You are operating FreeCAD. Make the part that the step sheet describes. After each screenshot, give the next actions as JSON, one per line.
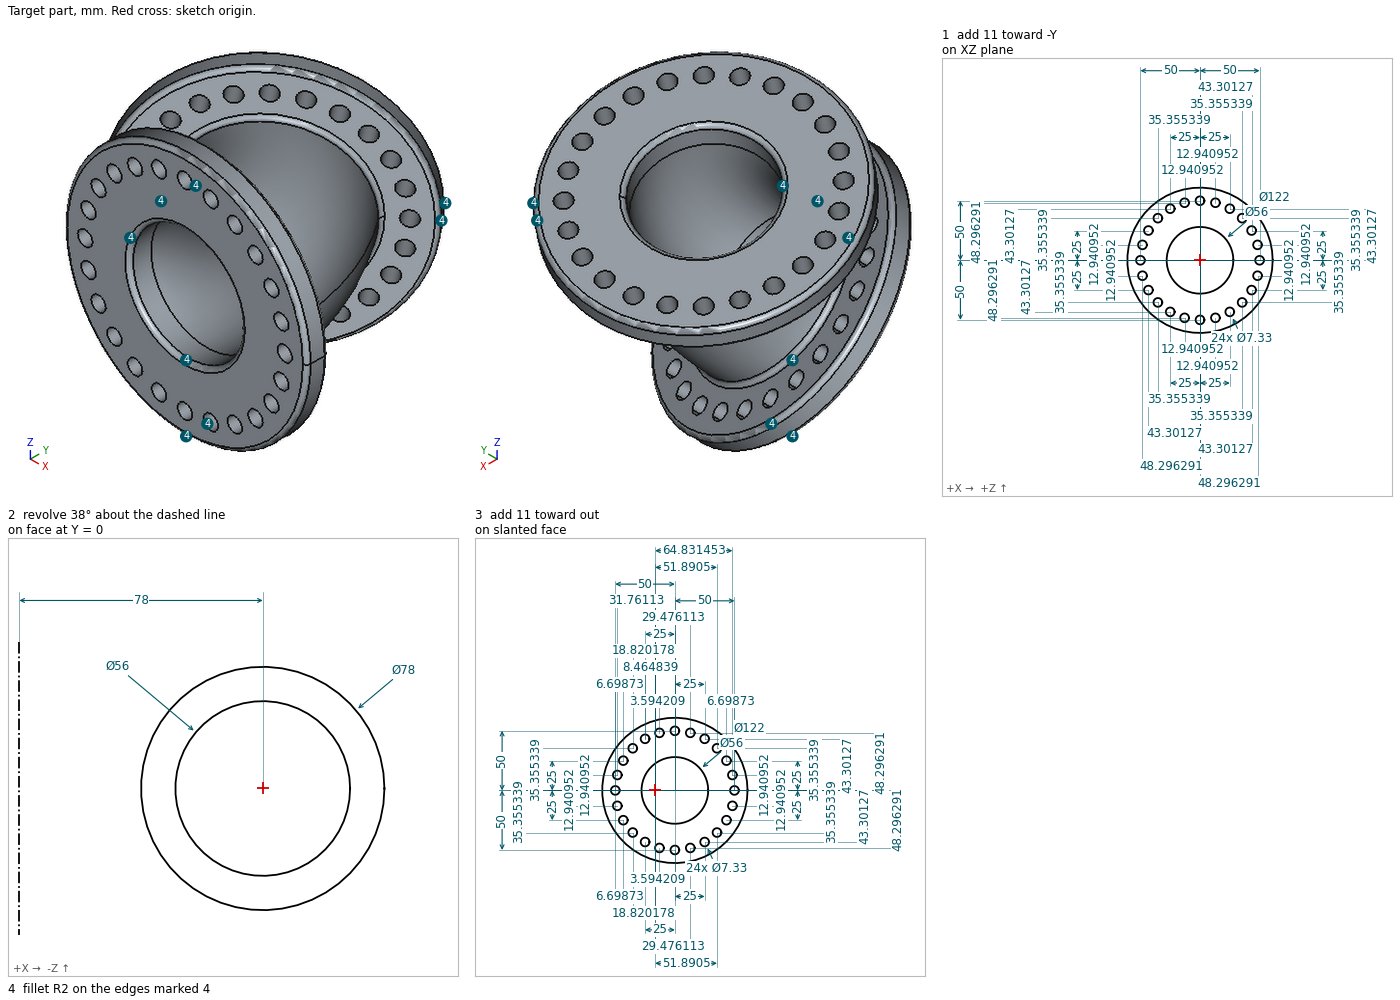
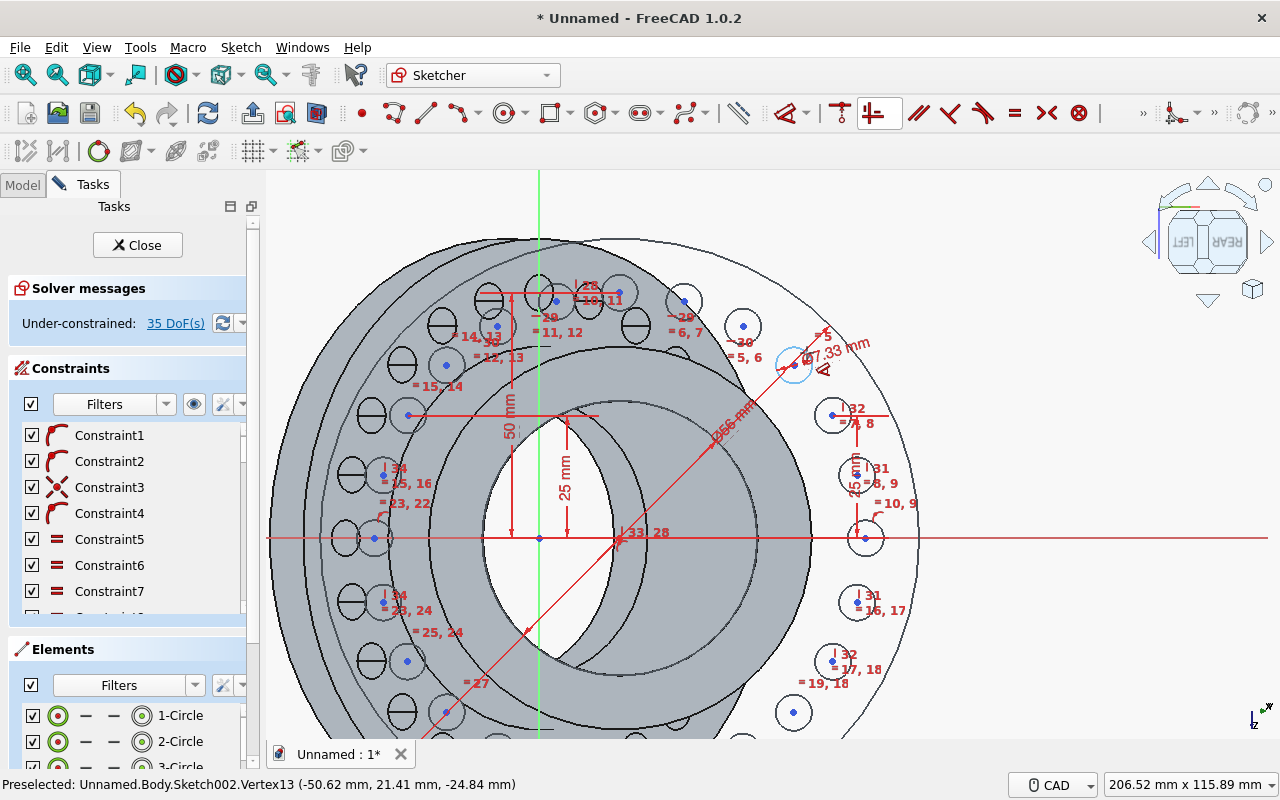
{"action": "left_click", "coordinate": [822, 523]}
{"action": "left_click", "coordinate": [626, 504]}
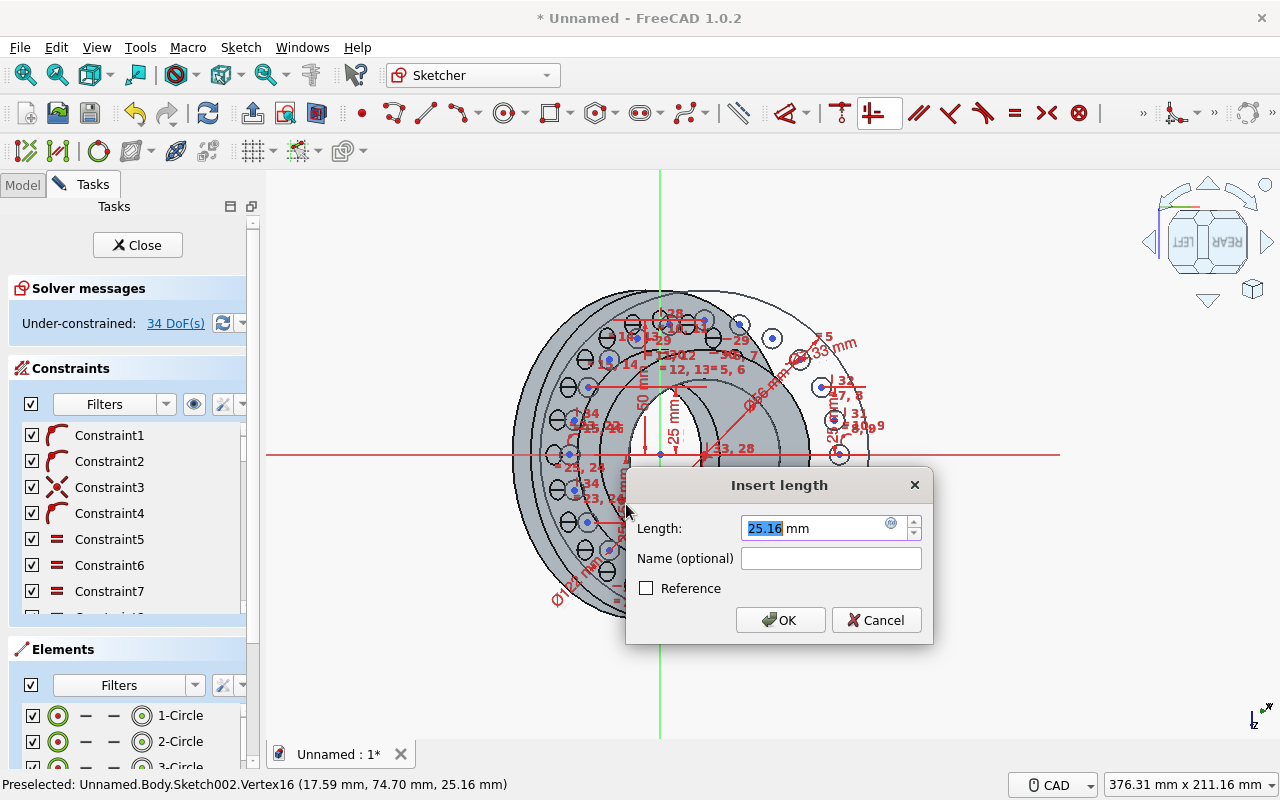
{"action": "type", "text": "25"}
{"action": "key", "text": "Return"}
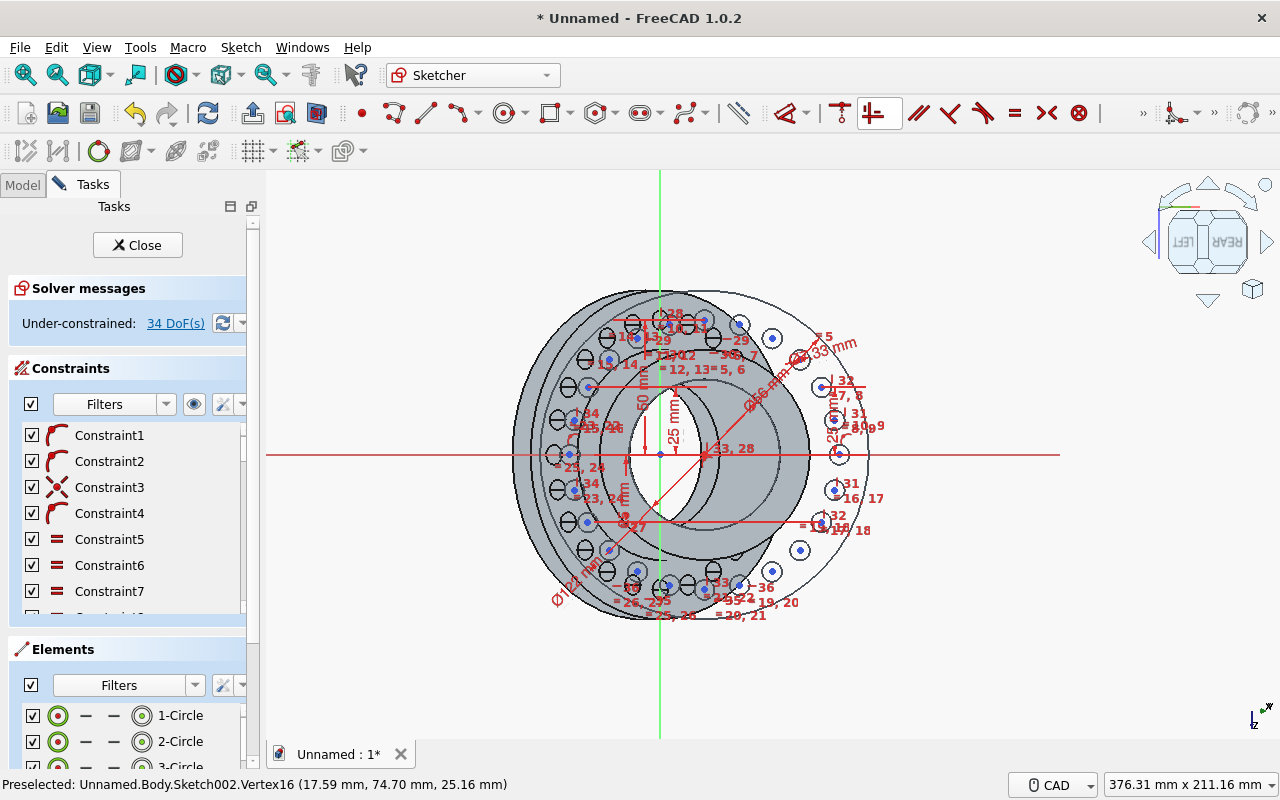
{"action": "left_click", "coordinate": [704, 590]}
{"action": "left_click", "coordinate": [738, 491]}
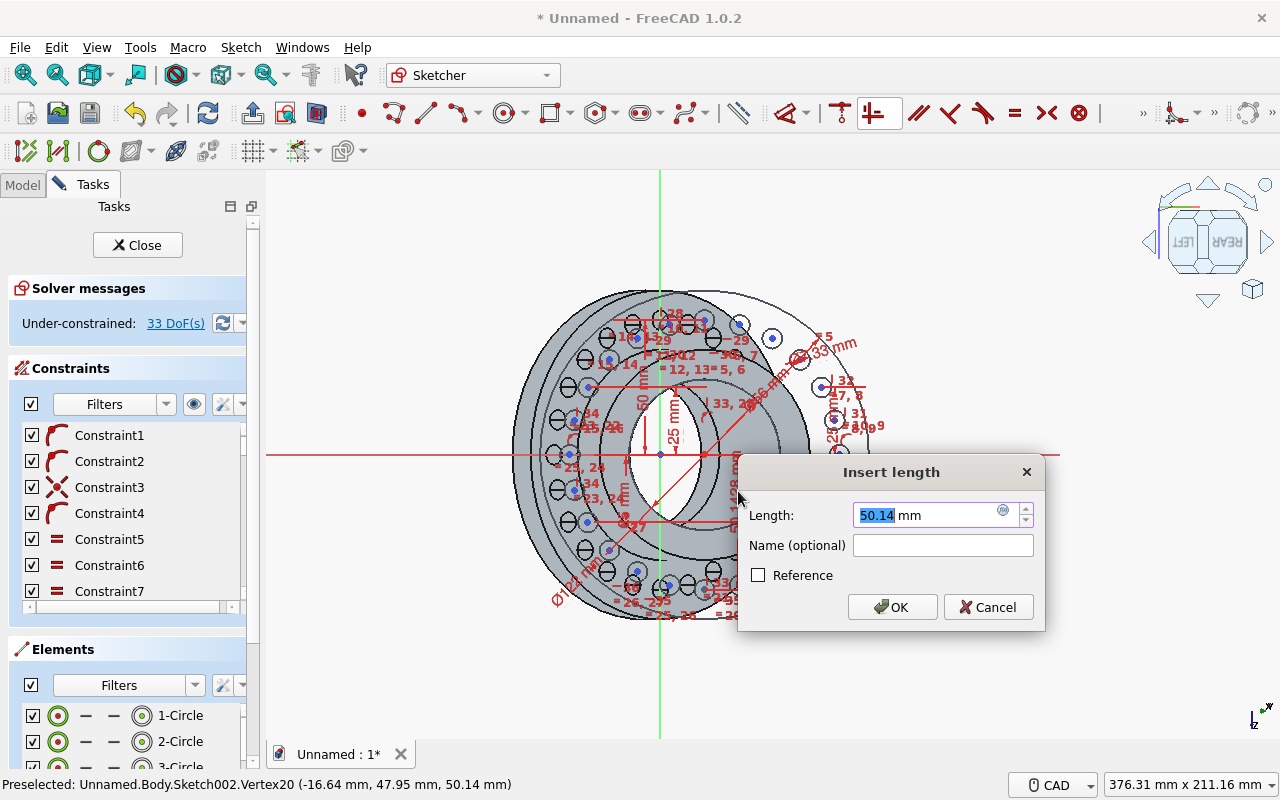
{"action": "type", "text": "50"}
{"action": "key", "text": "Return"}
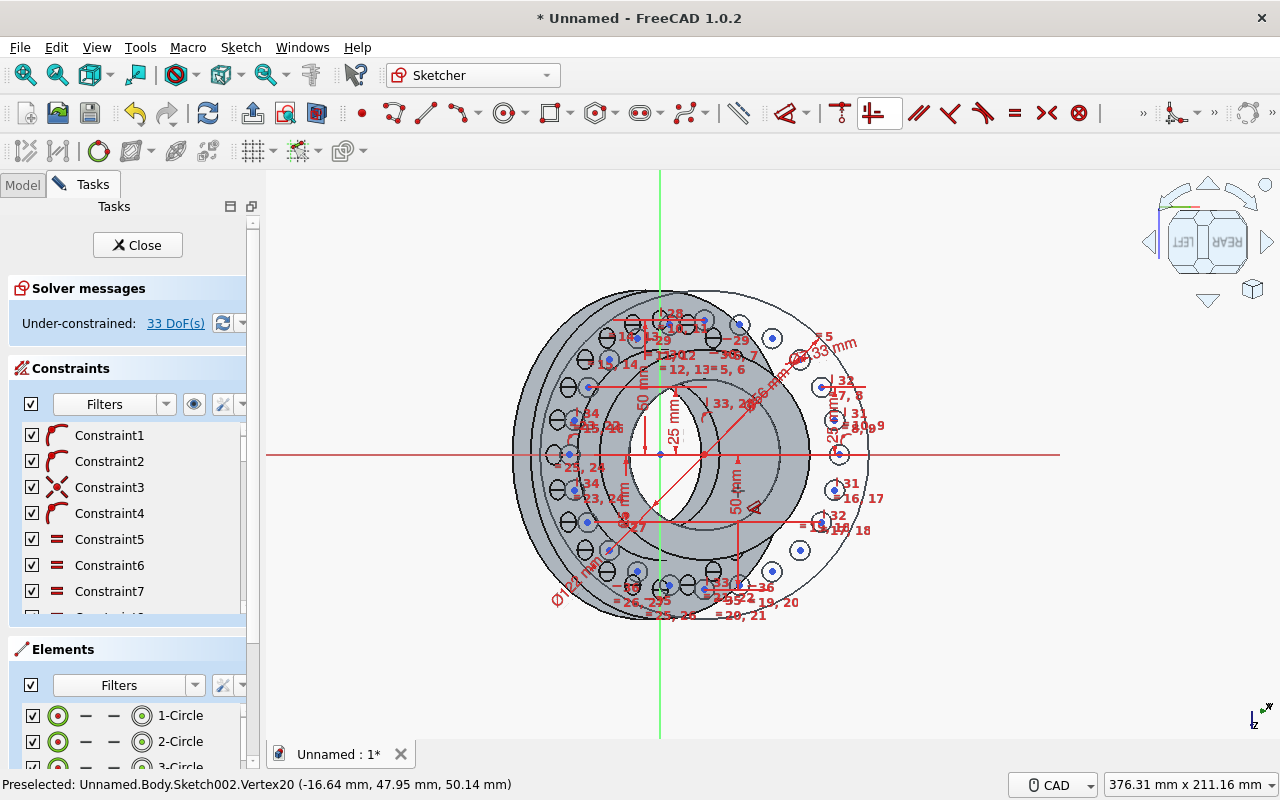
{"action": "left_click", "coordinate": [588, 522]}
{"action": "left_click", "coordinate": [530, 489]}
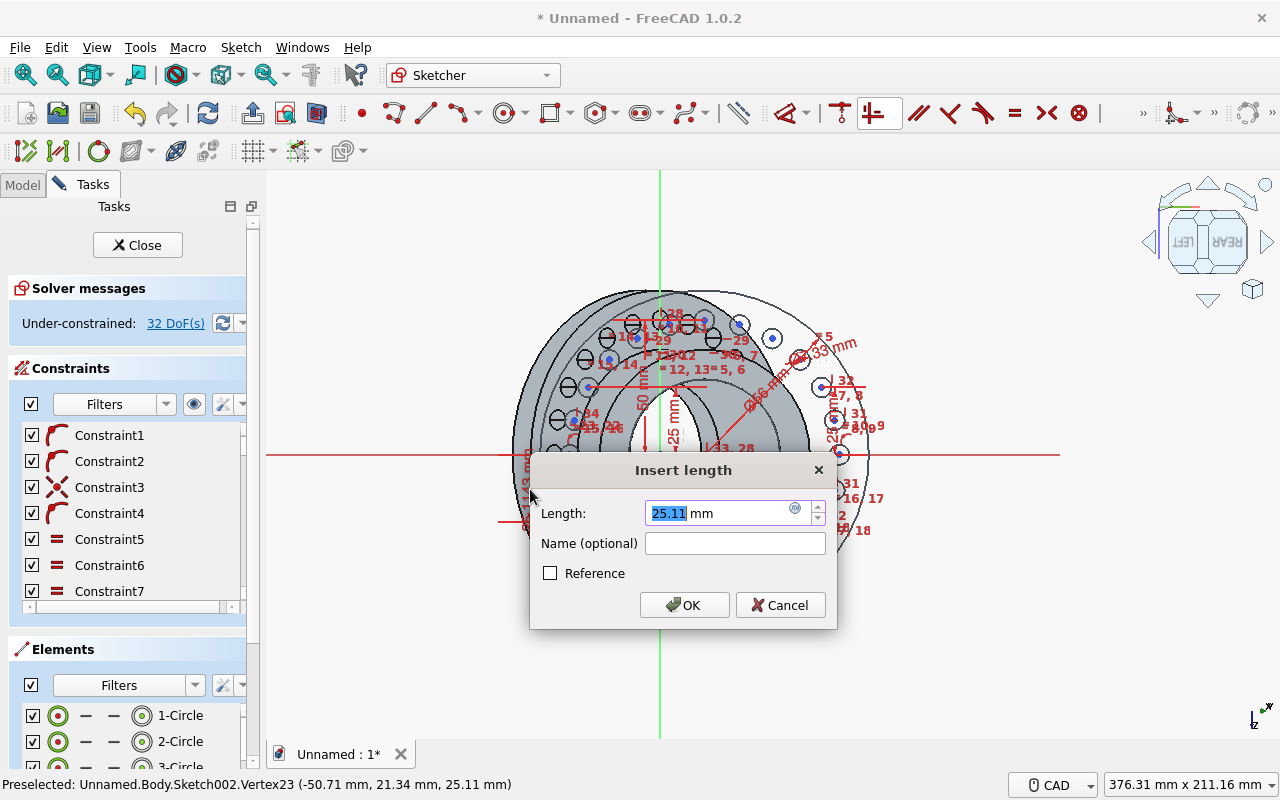
{"action": "type", "text": "25"}
{"action": "key", "text": "Return"}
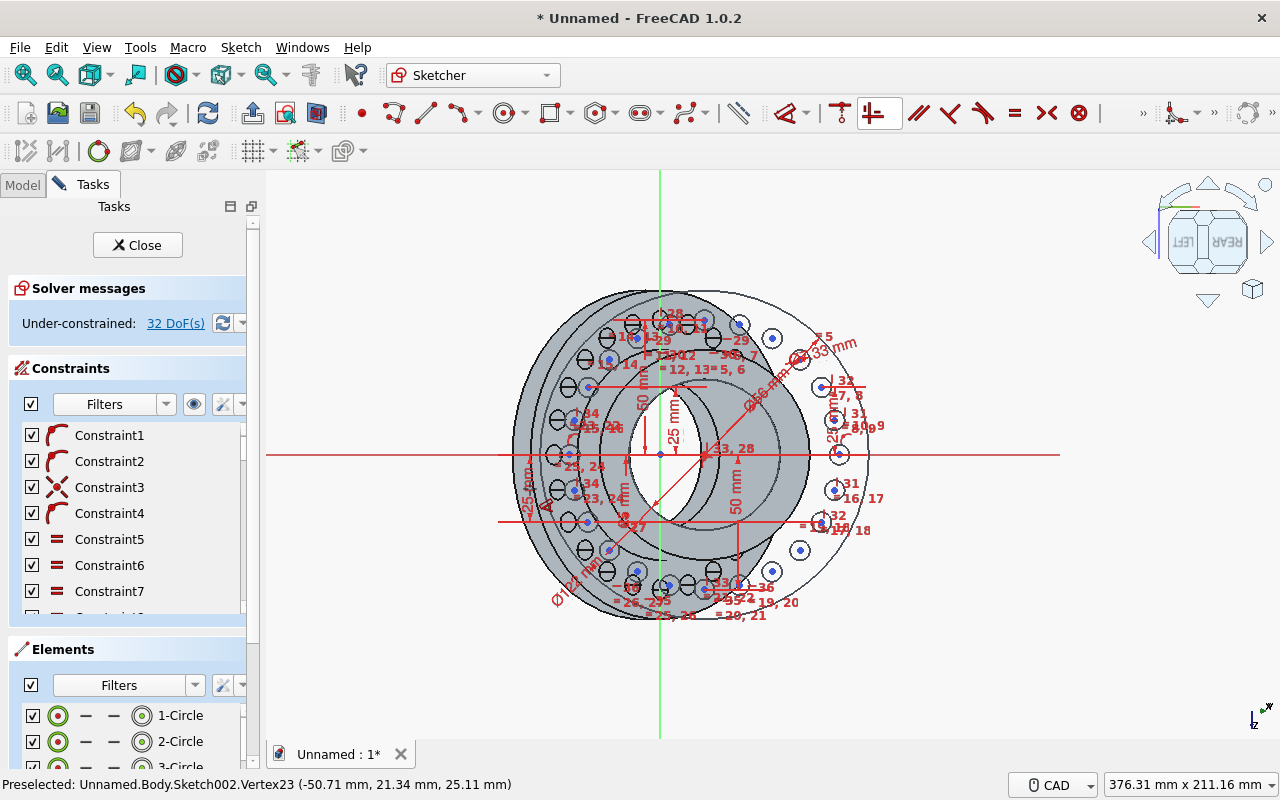
{"action": "left_click", "coordinate": [704, 455]}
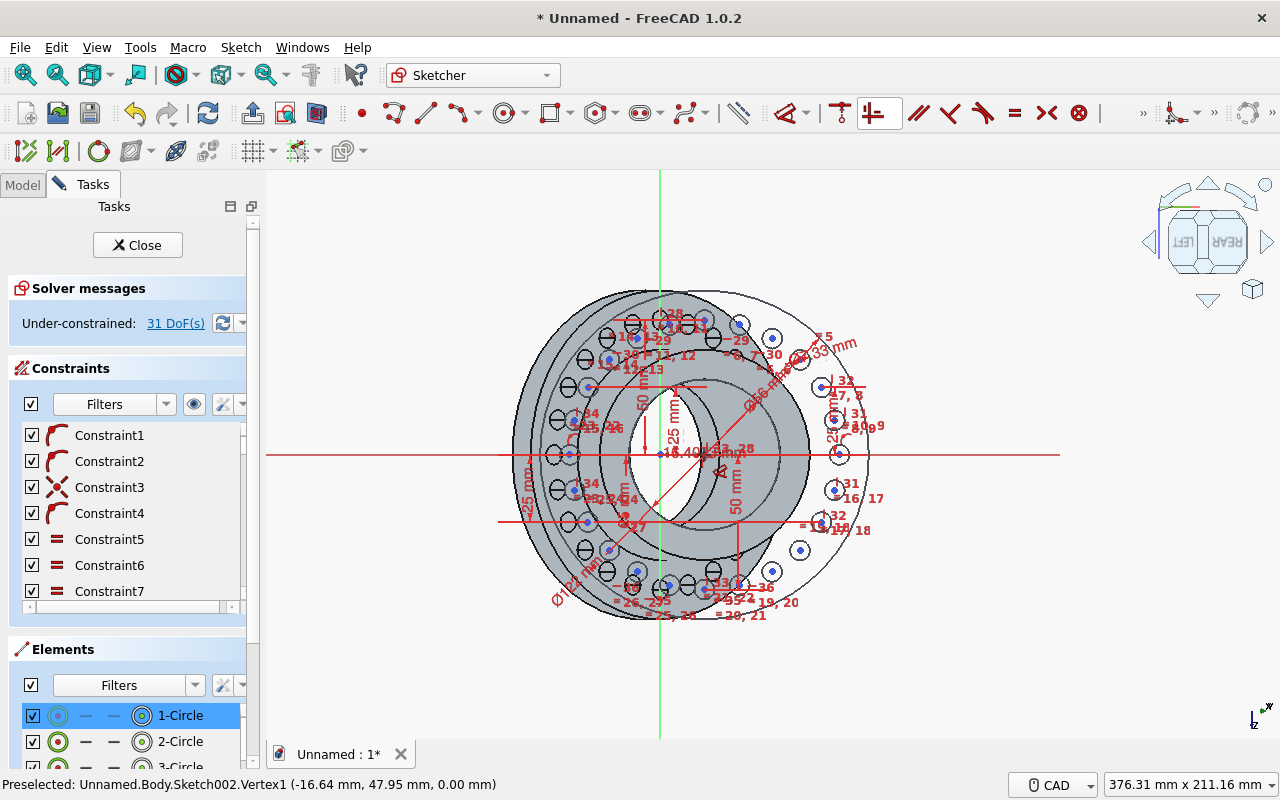
{"action": "left_click", "coordinate": [772, 339]}
{"action": "left_click", "coordinate": [723, 305]}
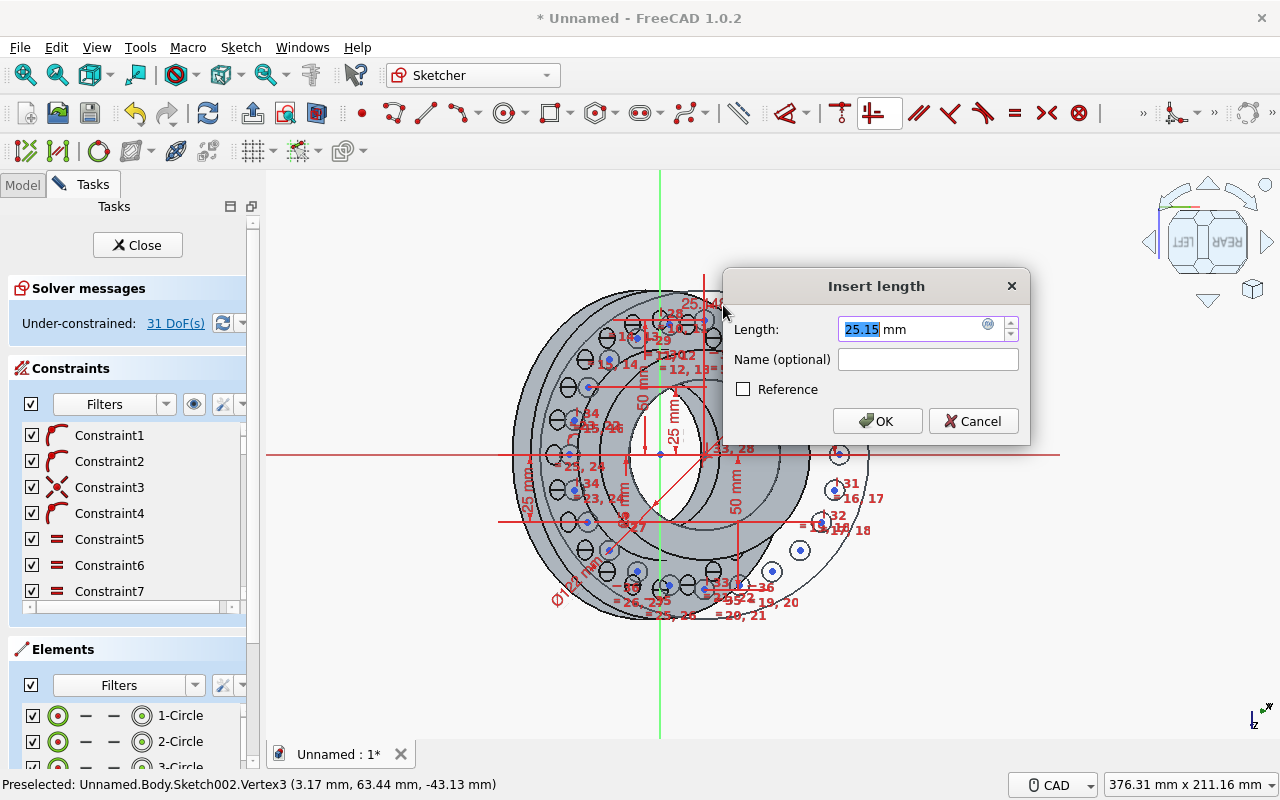
{"action": "type", "text": "25"}
{"action": "key", "text": "Return"}